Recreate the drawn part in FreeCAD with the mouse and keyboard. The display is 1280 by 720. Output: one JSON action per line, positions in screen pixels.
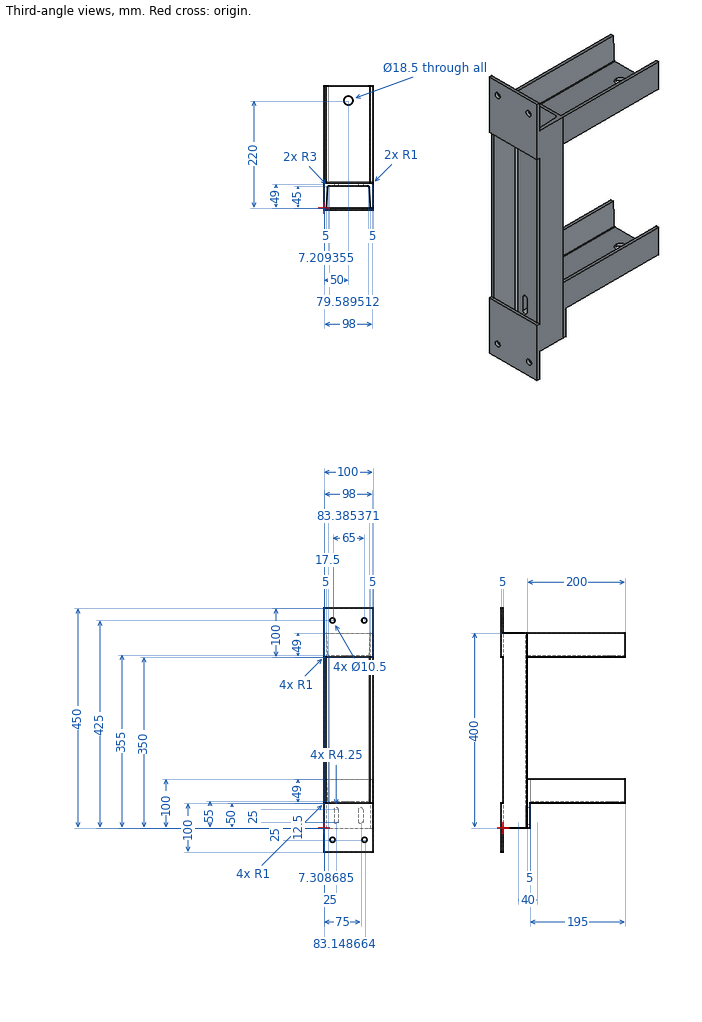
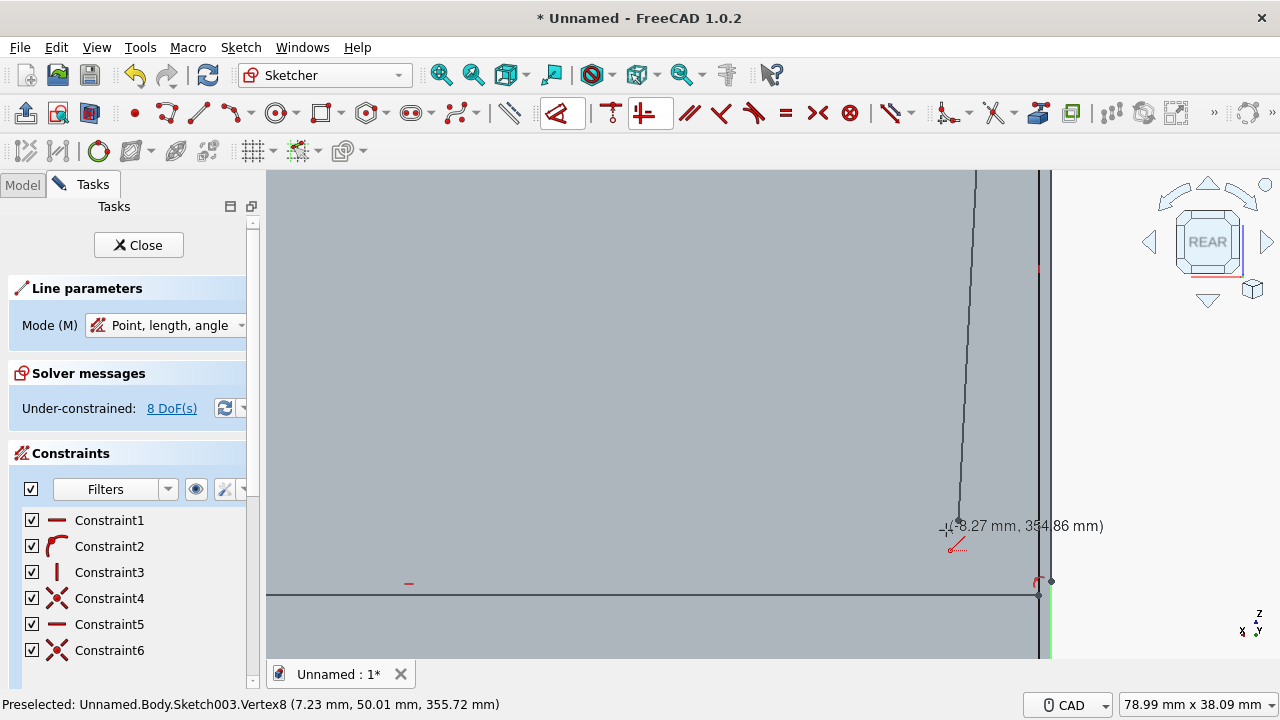
{"action": "left_click", "coordinate": [945, 529]}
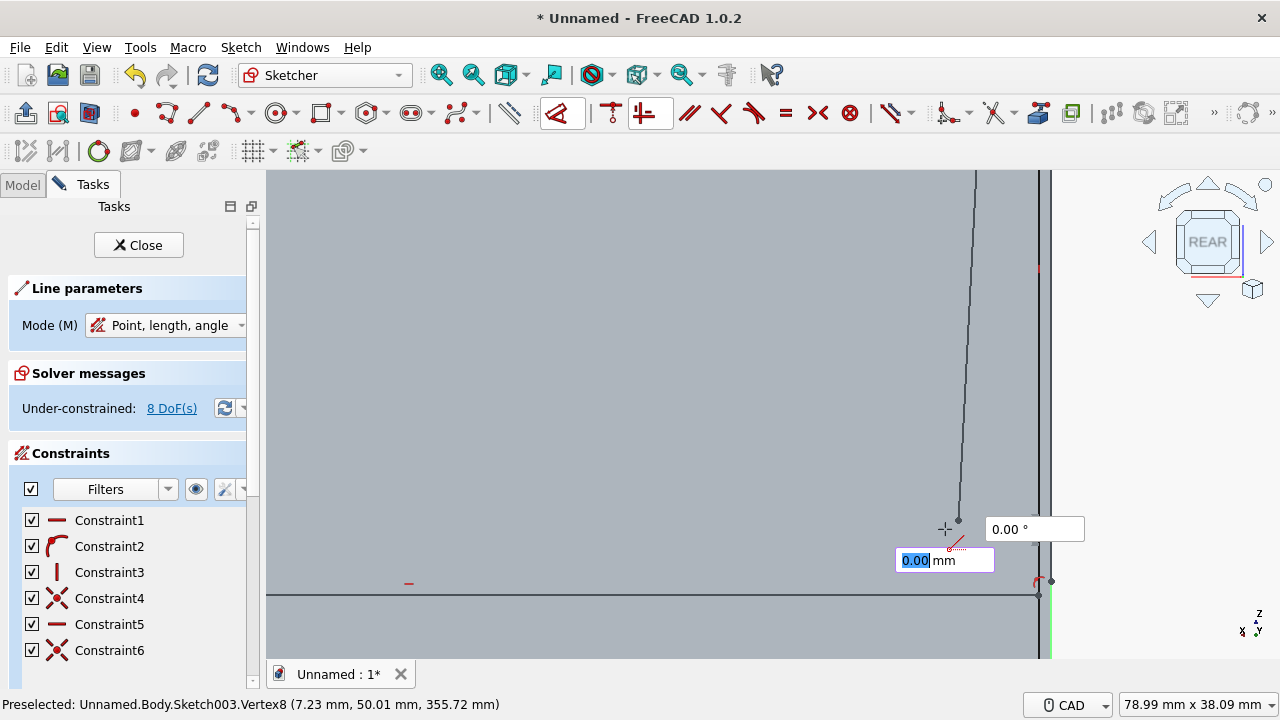
{"action": "scroll", "coordinate": [945, 530], "scroll_direction": "down", "scroll_amount": 4}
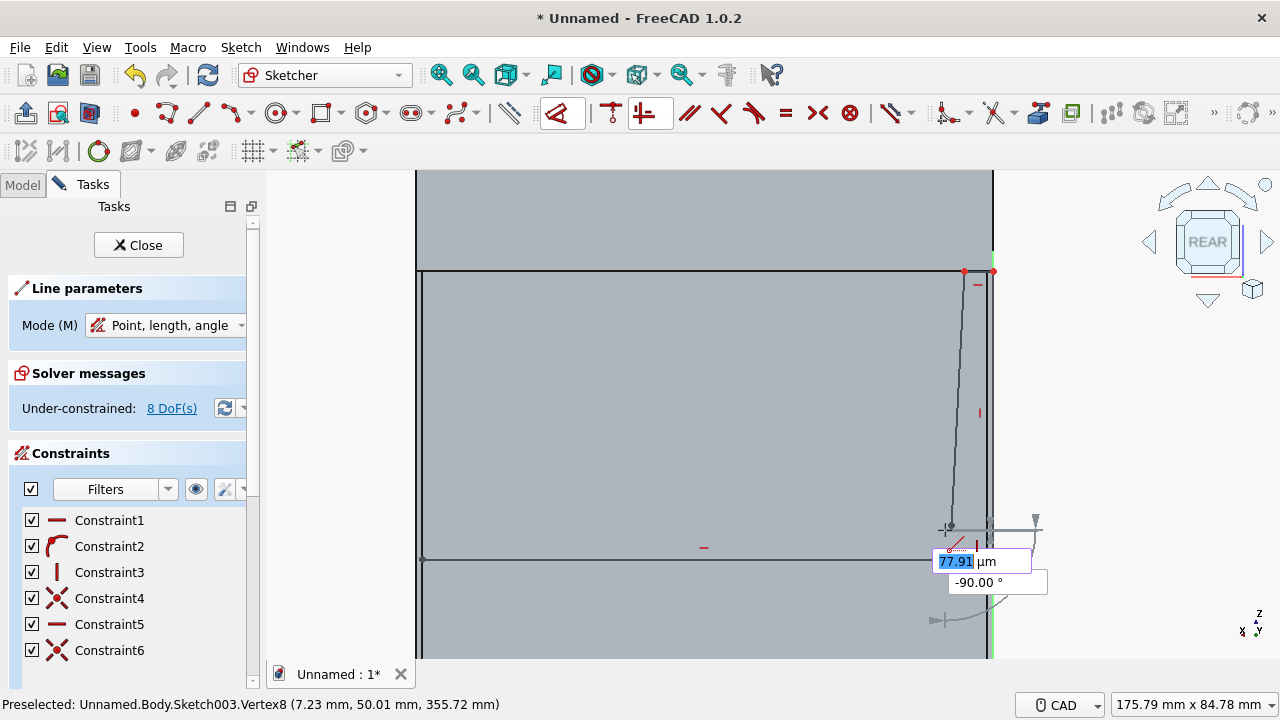
{"action": "left_click", "coordinate": [464, 530]}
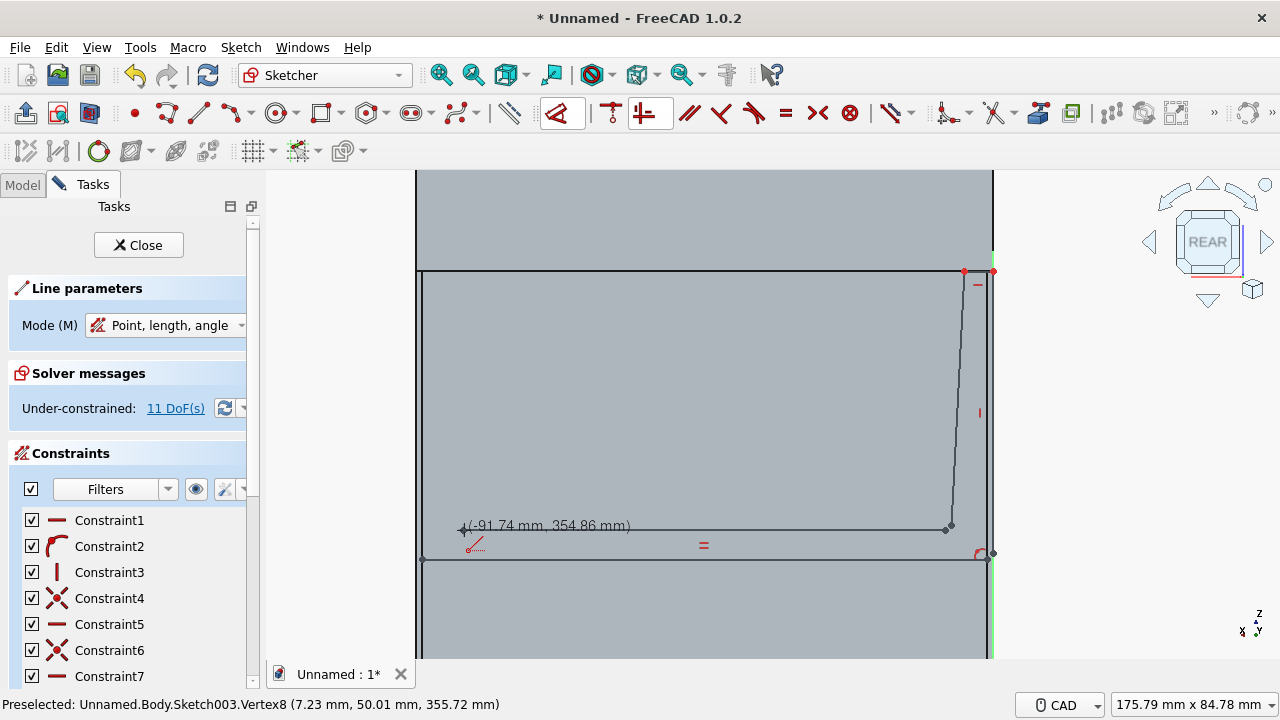
{"action": "left_click", "coordinate": [168, 114]}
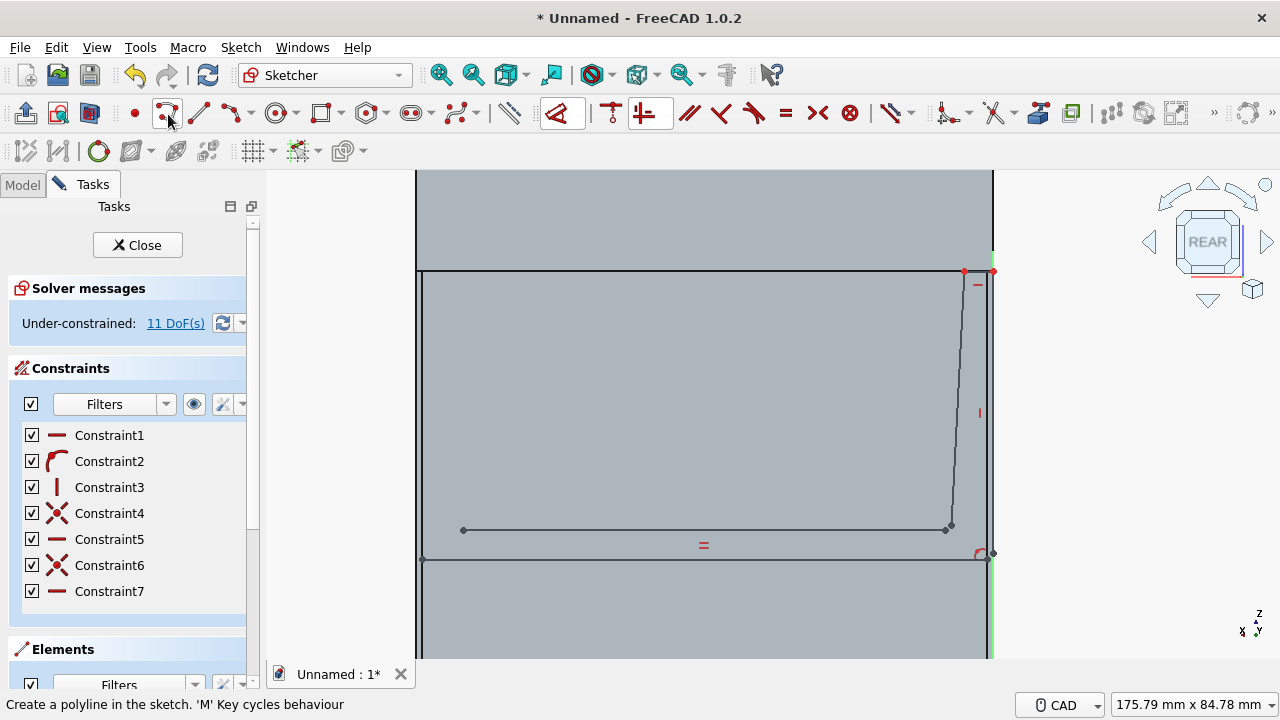
{"action": "scroll", "coordinate": [459, 525], "scroll_direction": "up", "scroll_amount": 4}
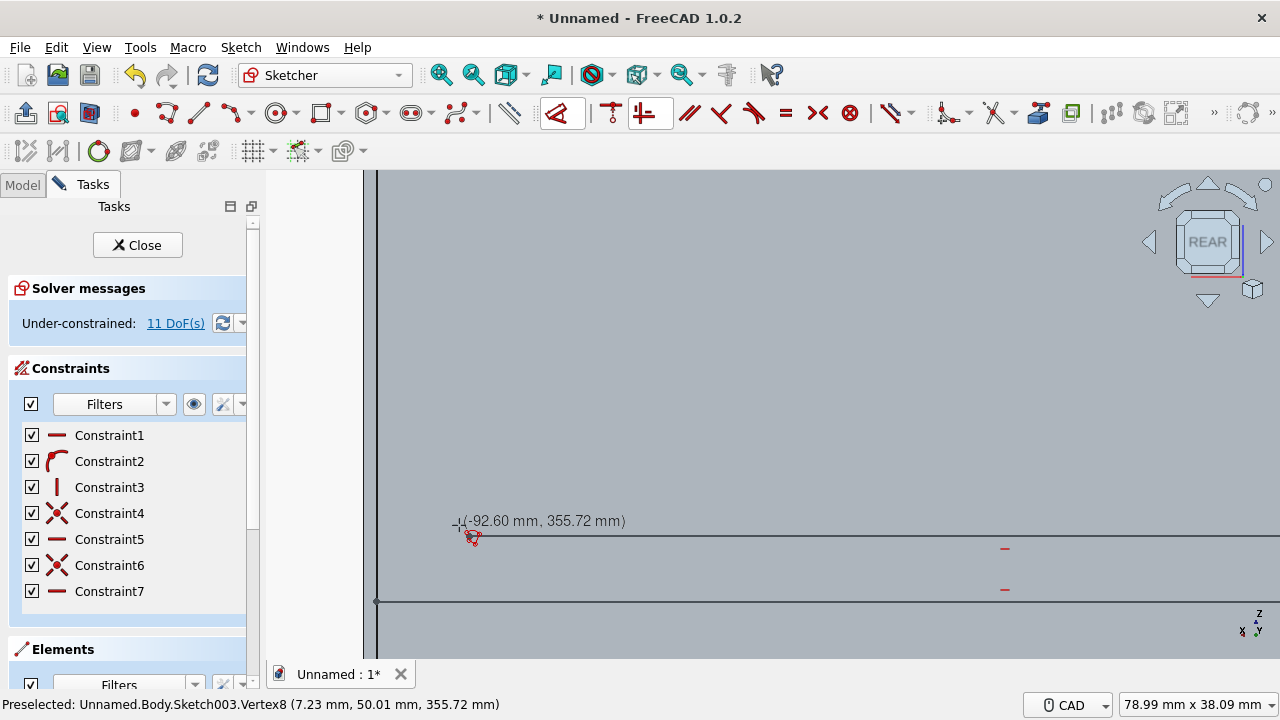
{"action": "left_click", "coordinate": [458, 523]}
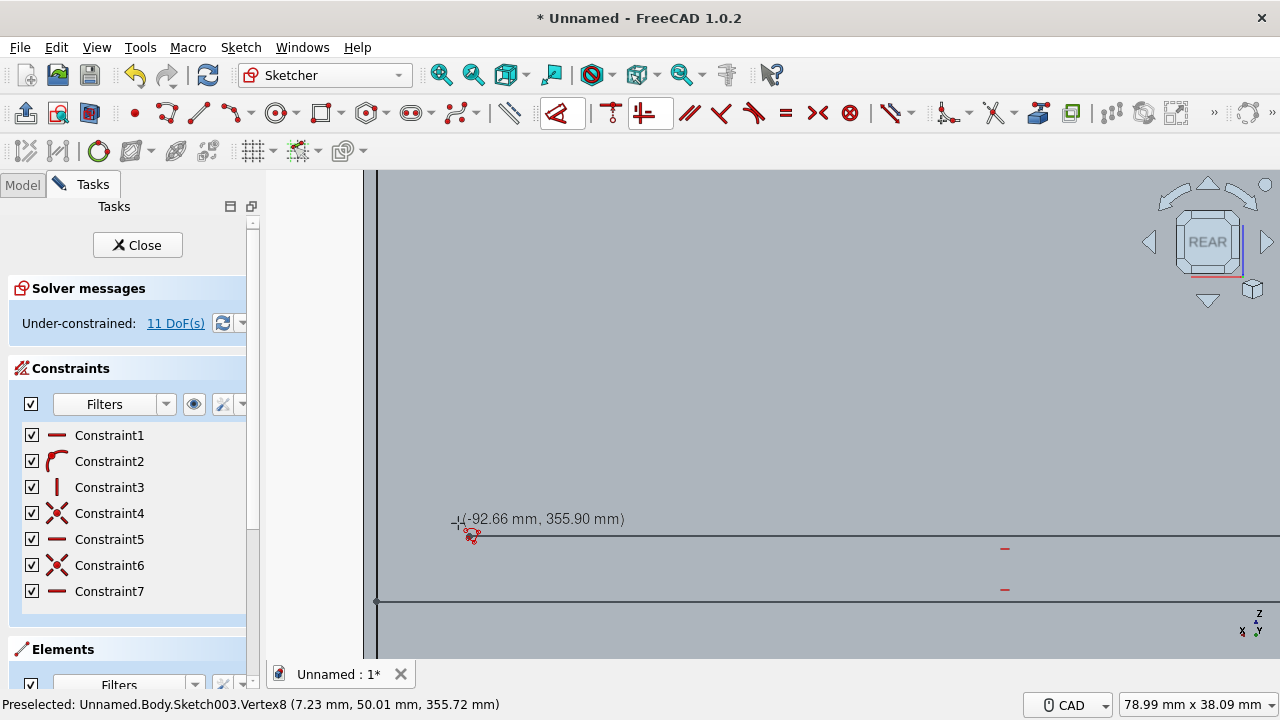
{"action": "scroll", "coordinate": [459, 525], "scroll_direction": "down", "scroll_amount": 4}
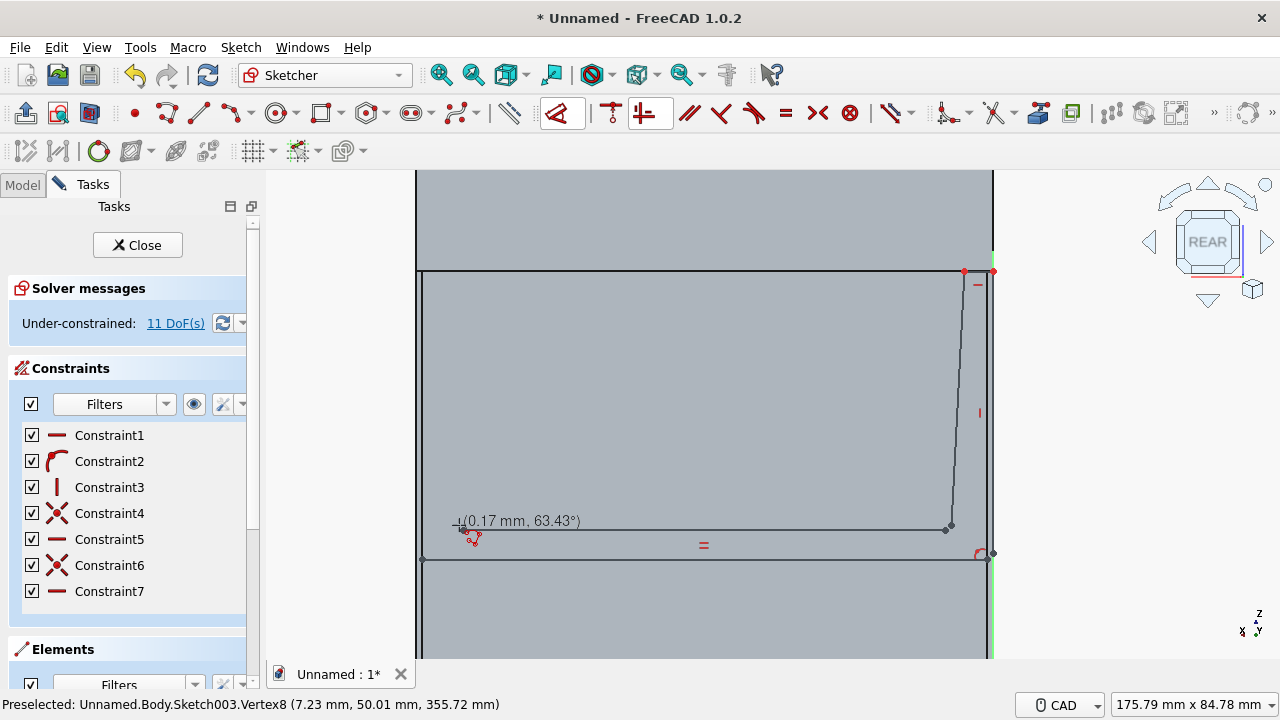
{"action": "left_click", "coordinate": [445, 271]}
{"action": "left_click", "coordinate": [416, 271]}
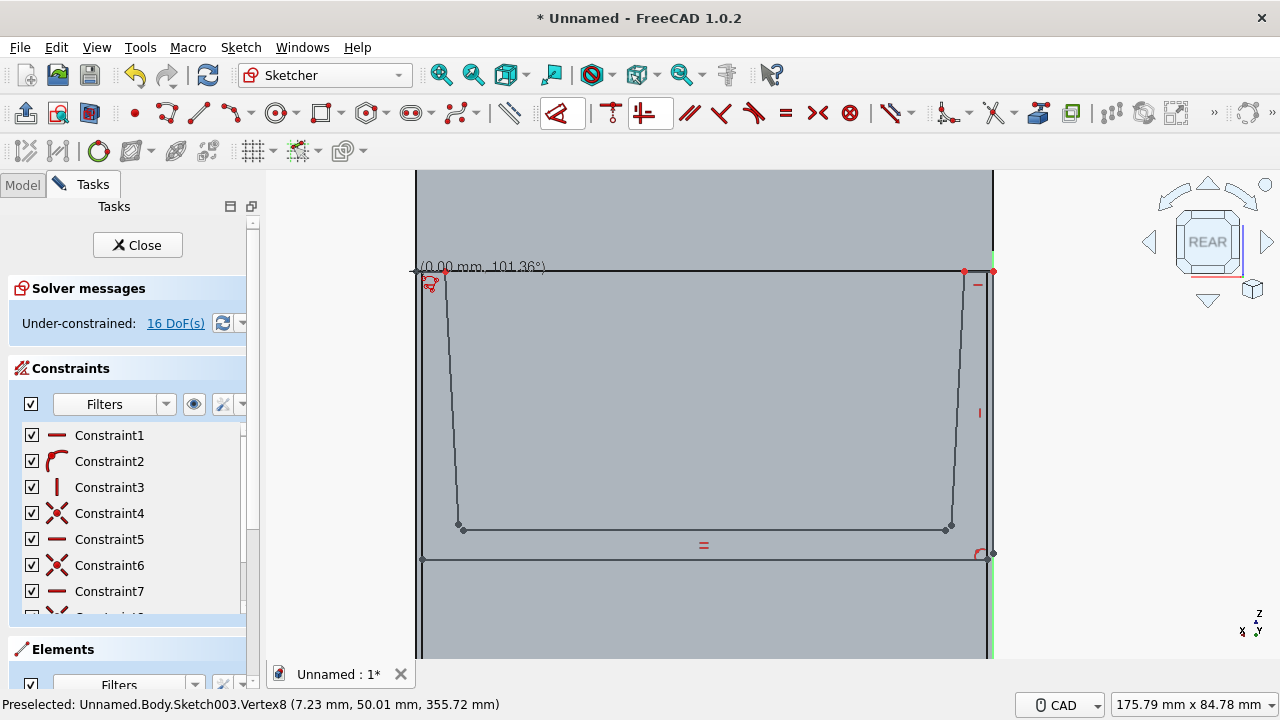
{"action": "scroll", "coordinate": [416, 553], "scroll_direction": "up", "scroll_amount": 4}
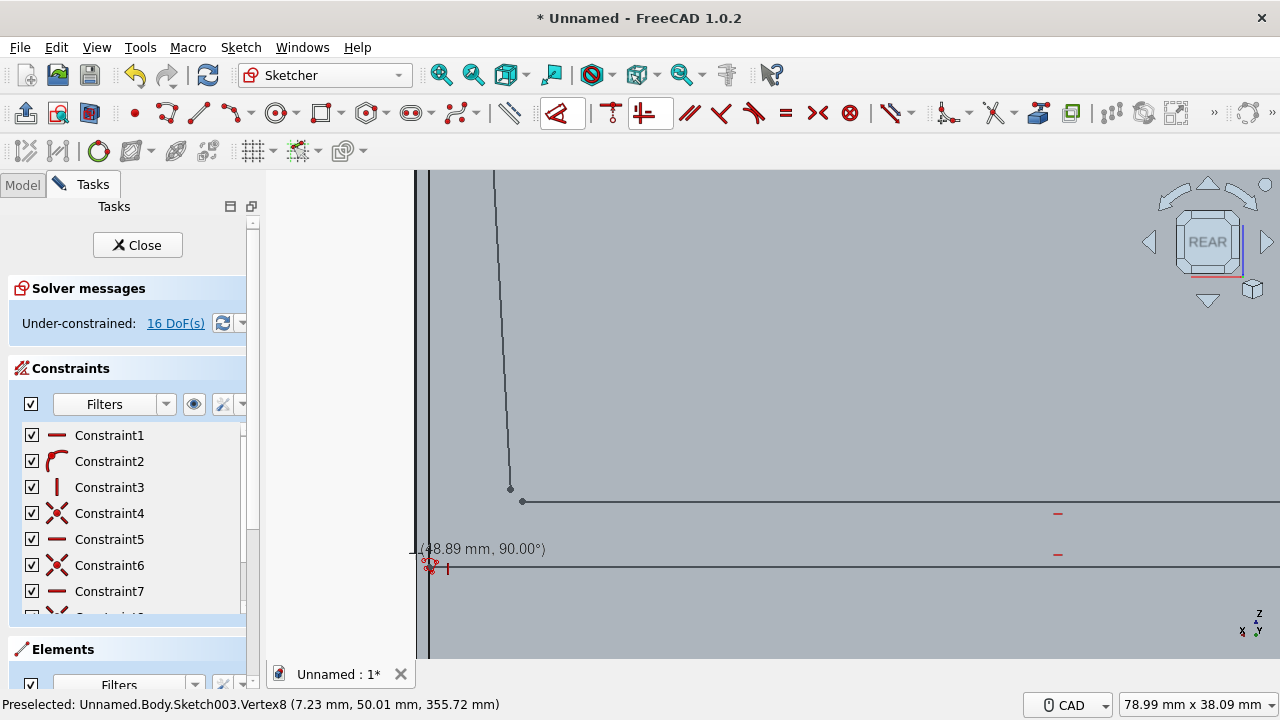
{"action": "left_click", "coordinate": [416, 553]}
{"action": "right_click", "coordinate": [416, 553]}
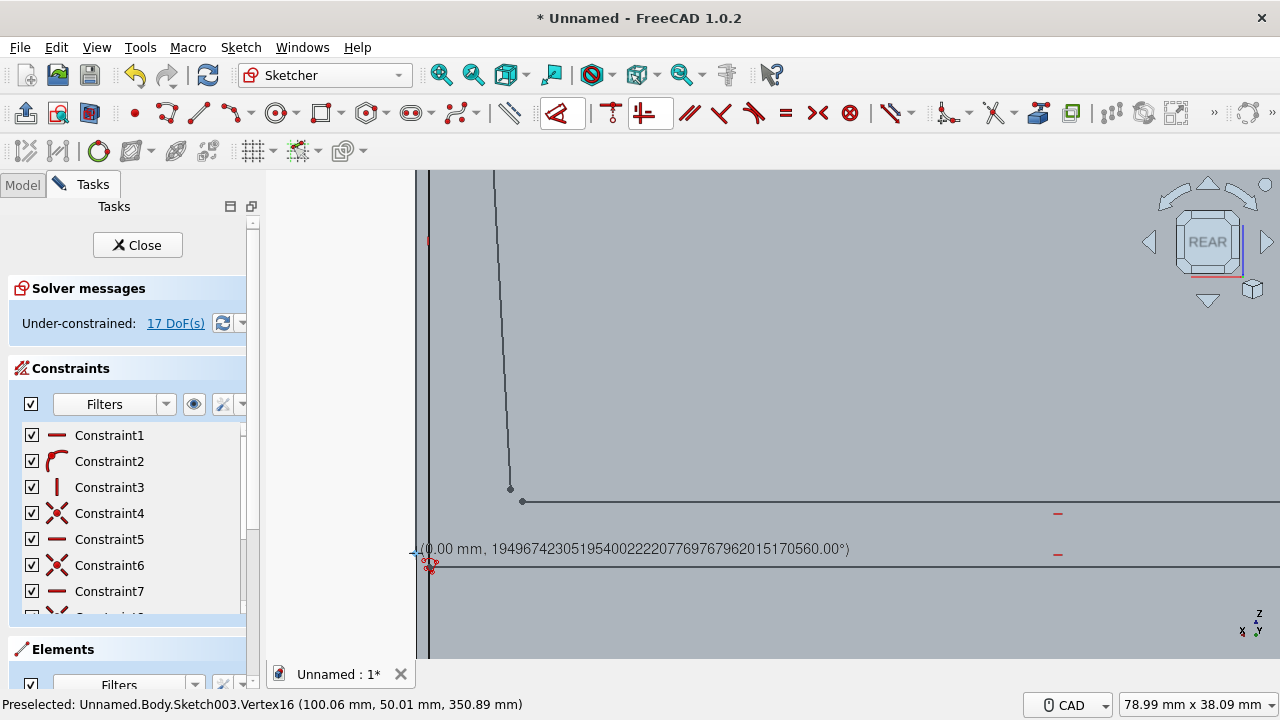
{"action": "left_click", "coordinate": [232, 114]}